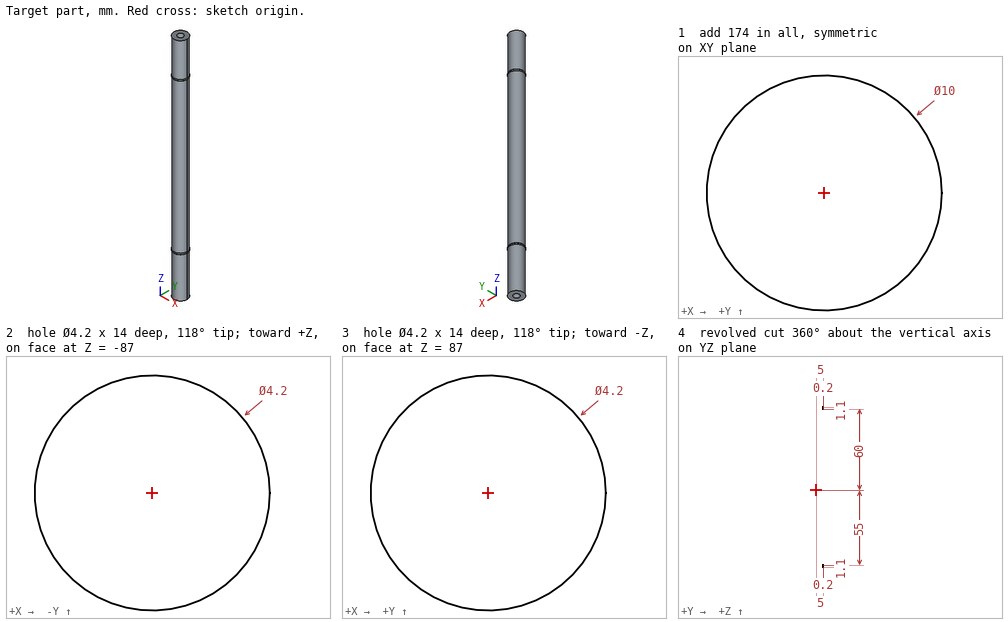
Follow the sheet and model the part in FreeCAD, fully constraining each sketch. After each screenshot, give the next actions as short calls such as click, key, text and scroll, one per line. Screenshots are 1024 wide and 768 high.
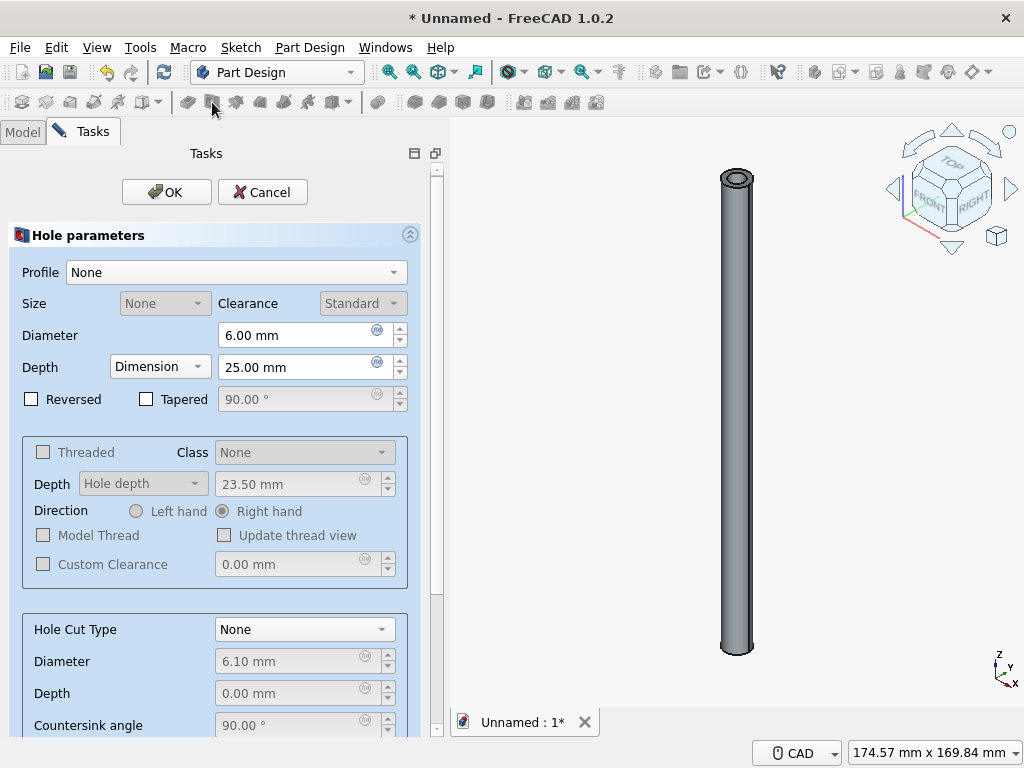
triple_click(305, 335)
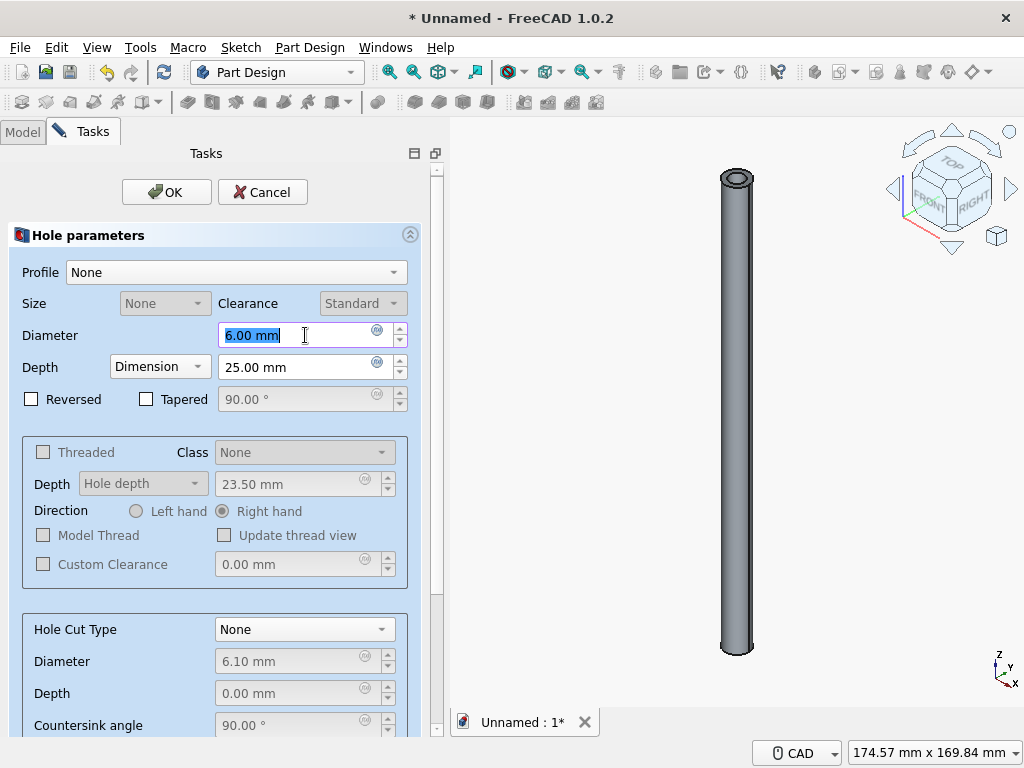
text(4.2)
key(Tab)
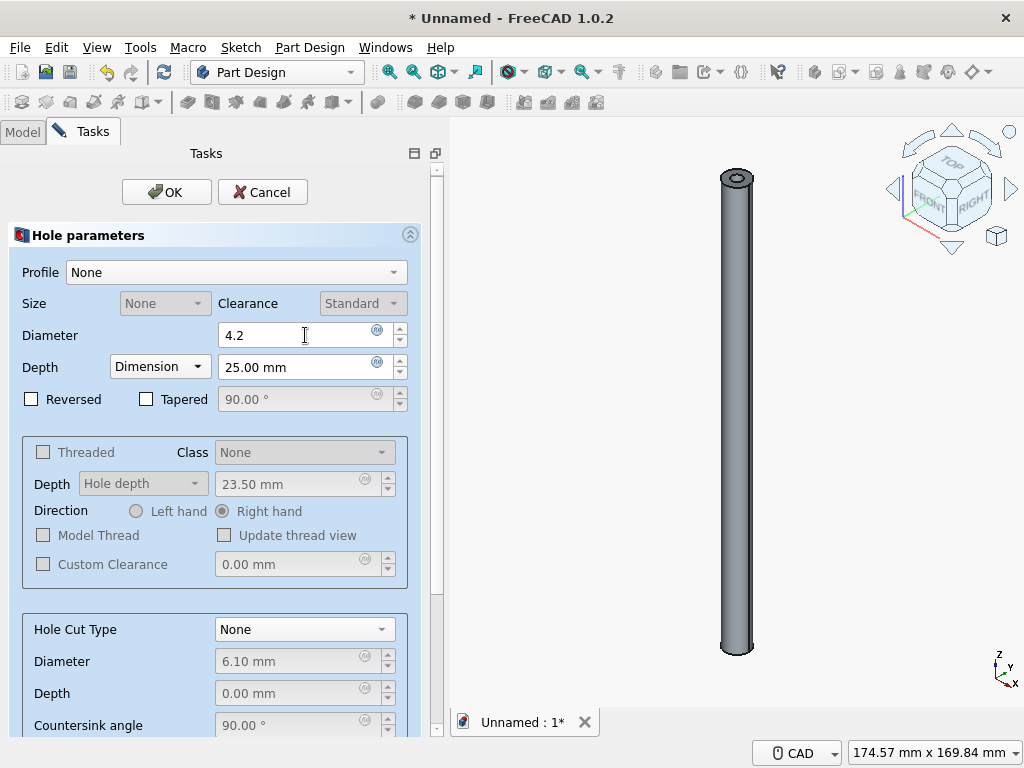
triple_click(305, 367)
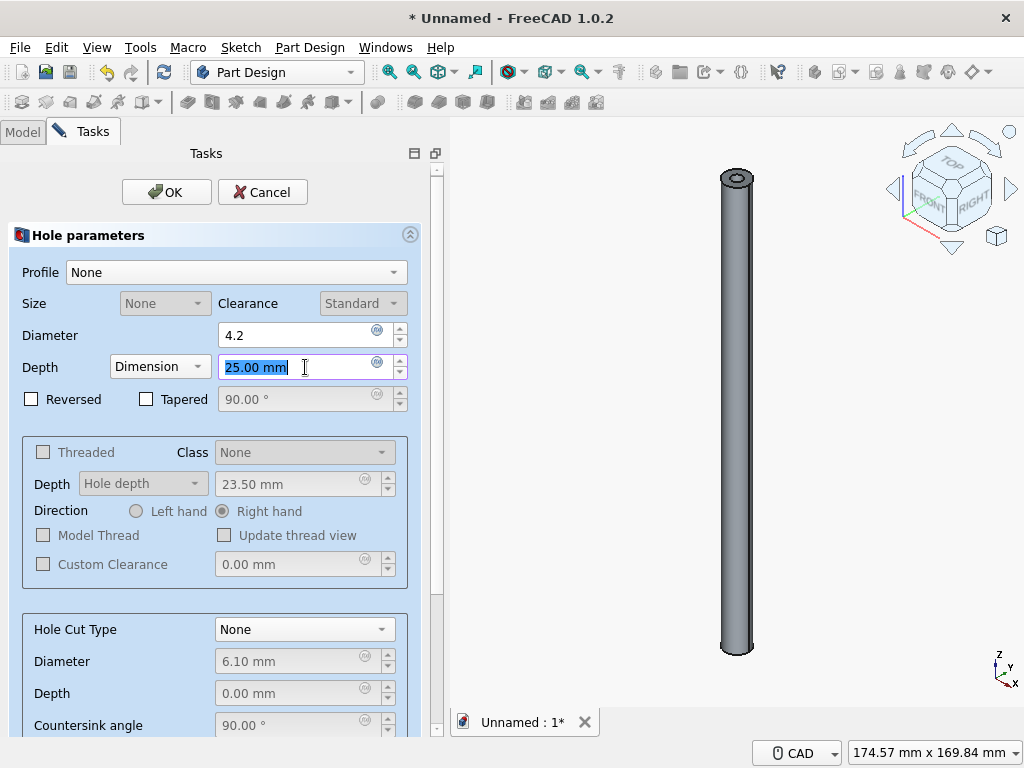
text(14)
key(Tab)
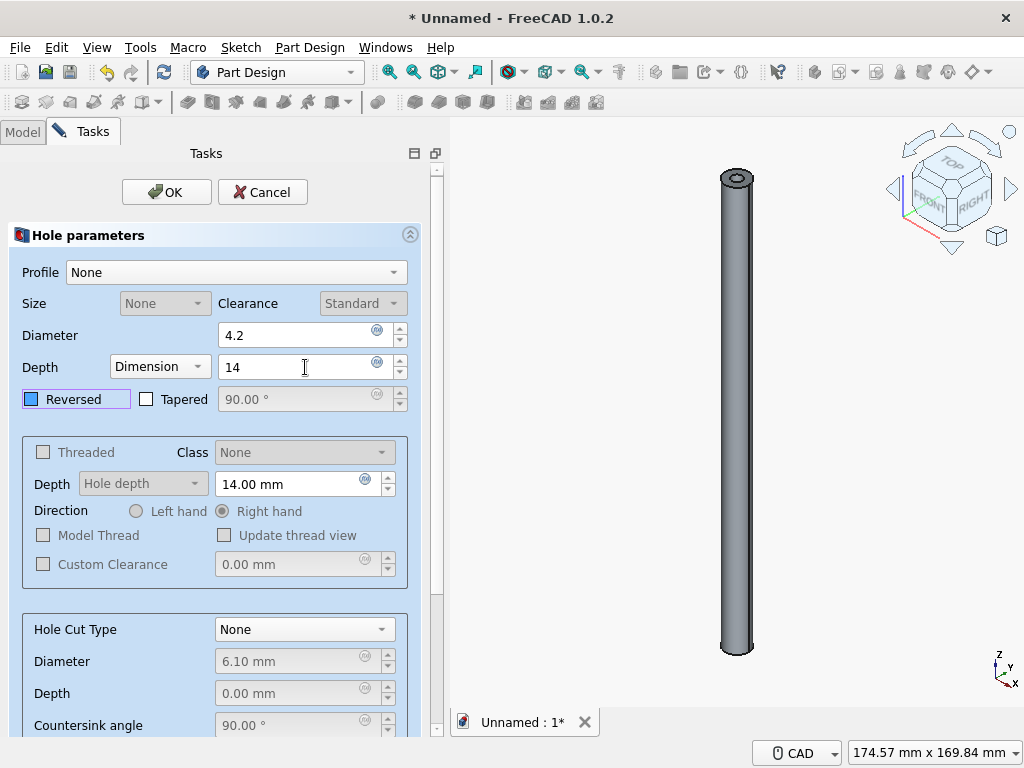
click(167, 192)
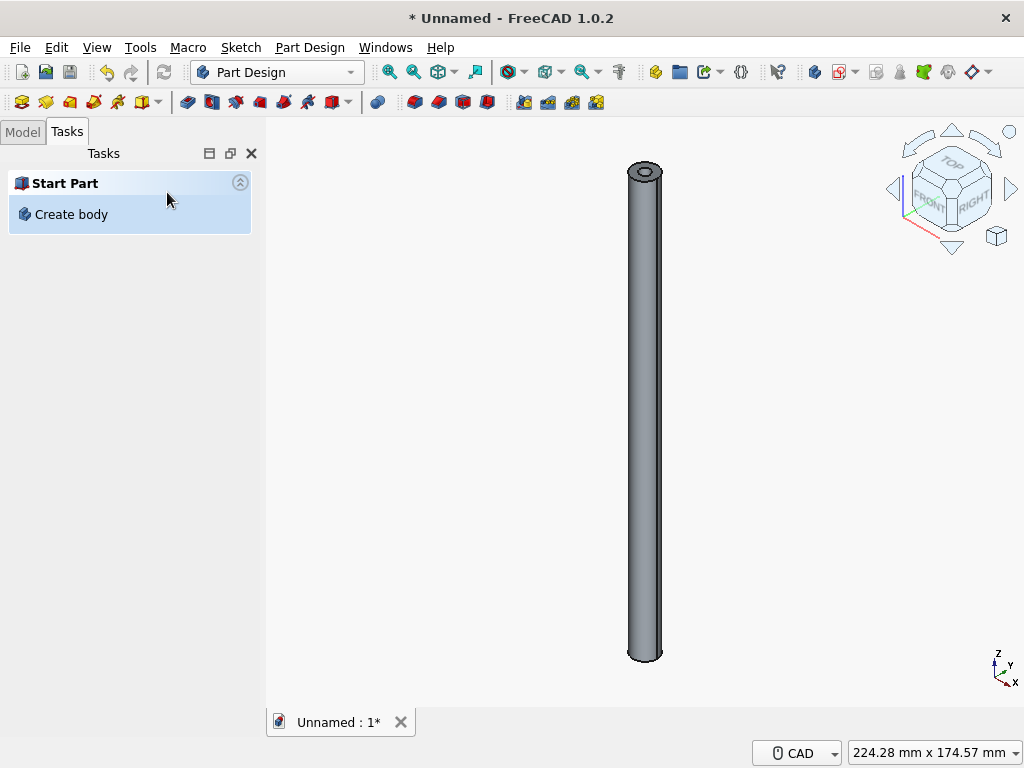
click(840, 72)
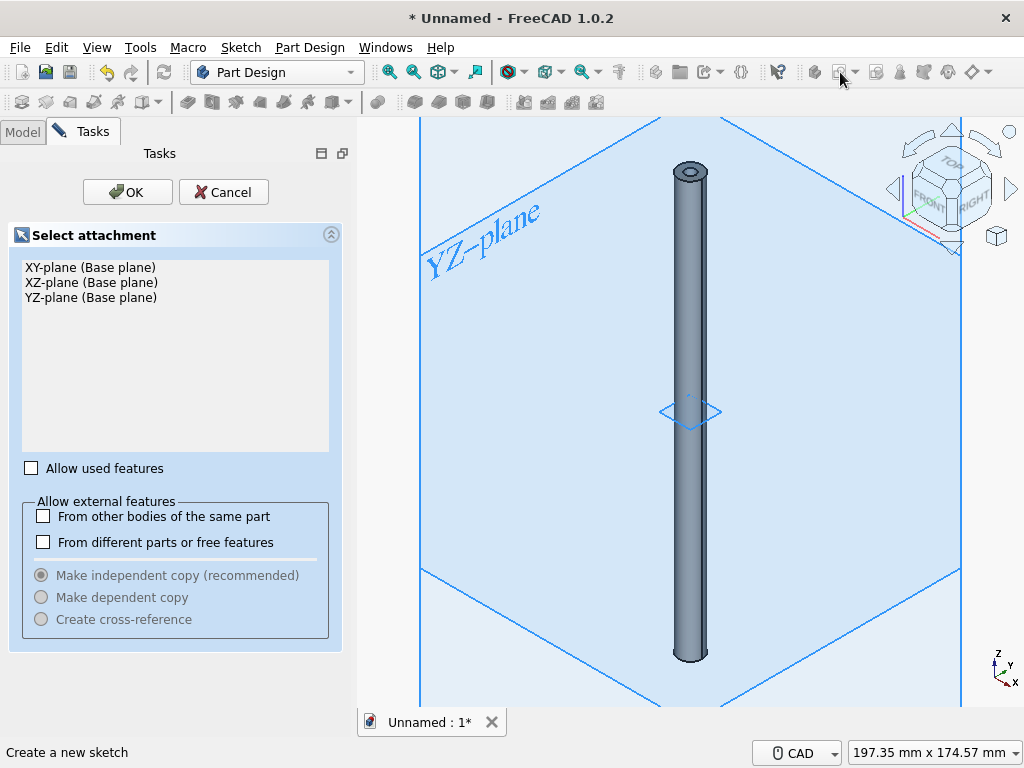
click(82, 298)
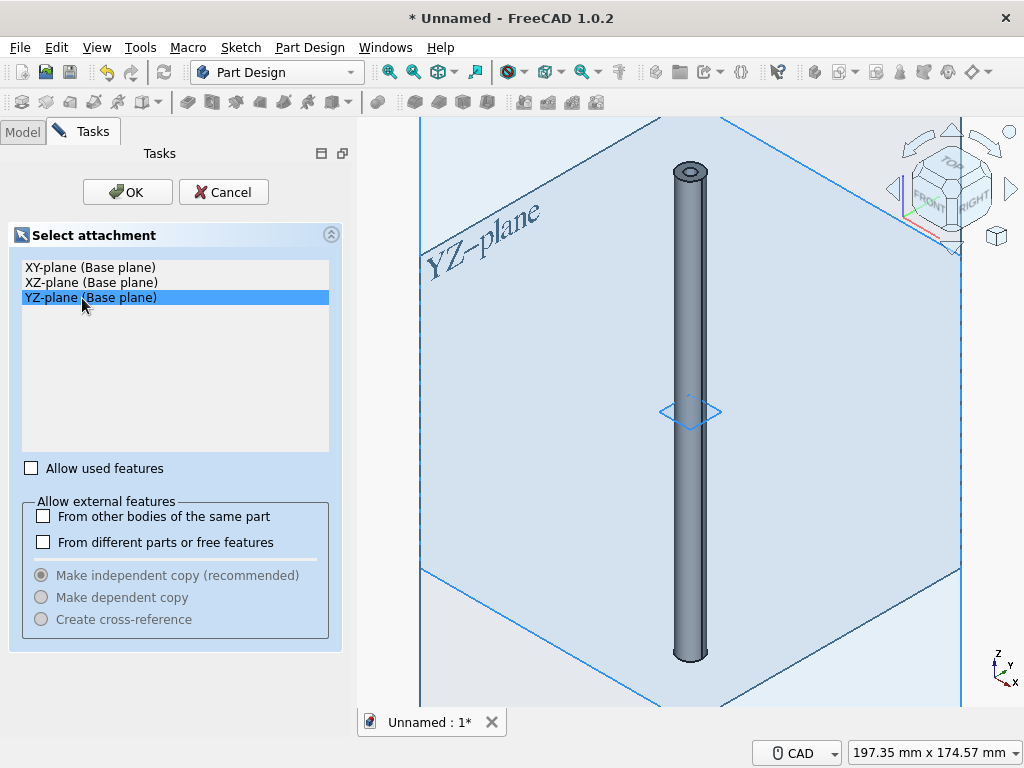
click(128, 192)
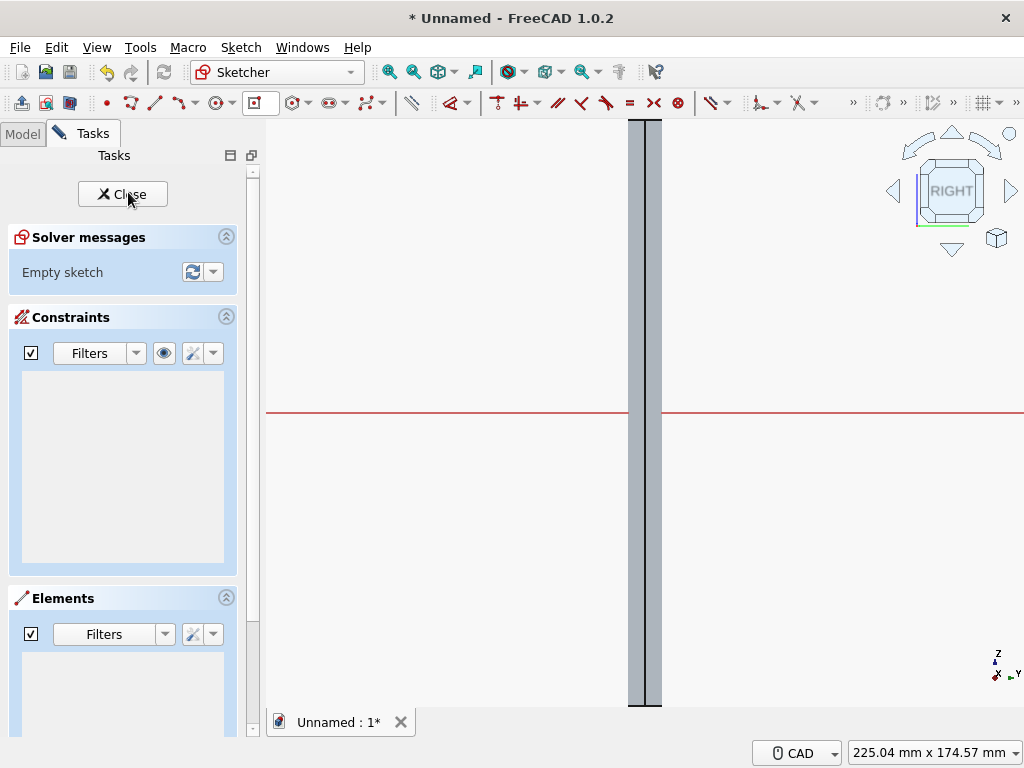
click(70, 104)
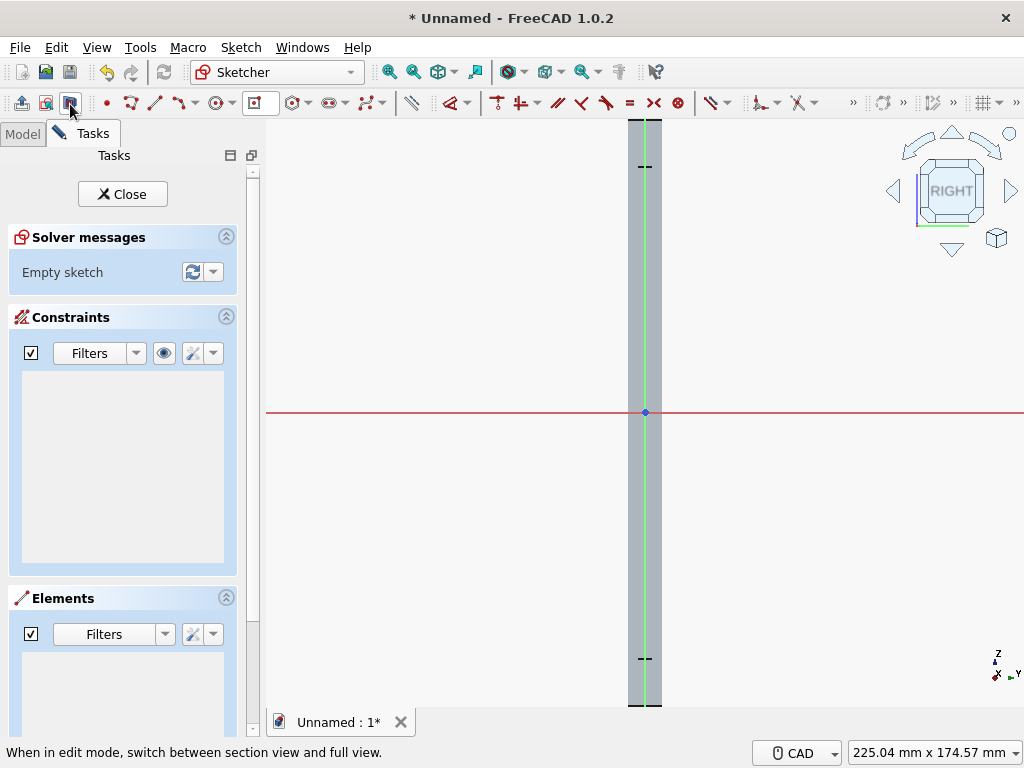
click(274, 104)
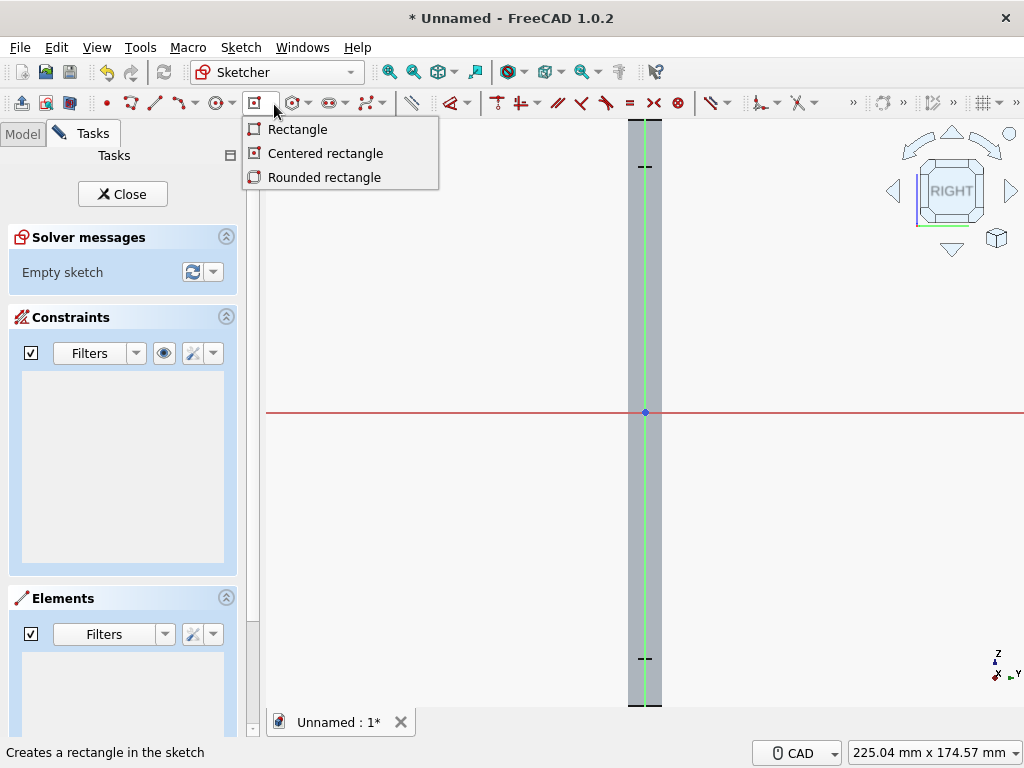
click(340, 129)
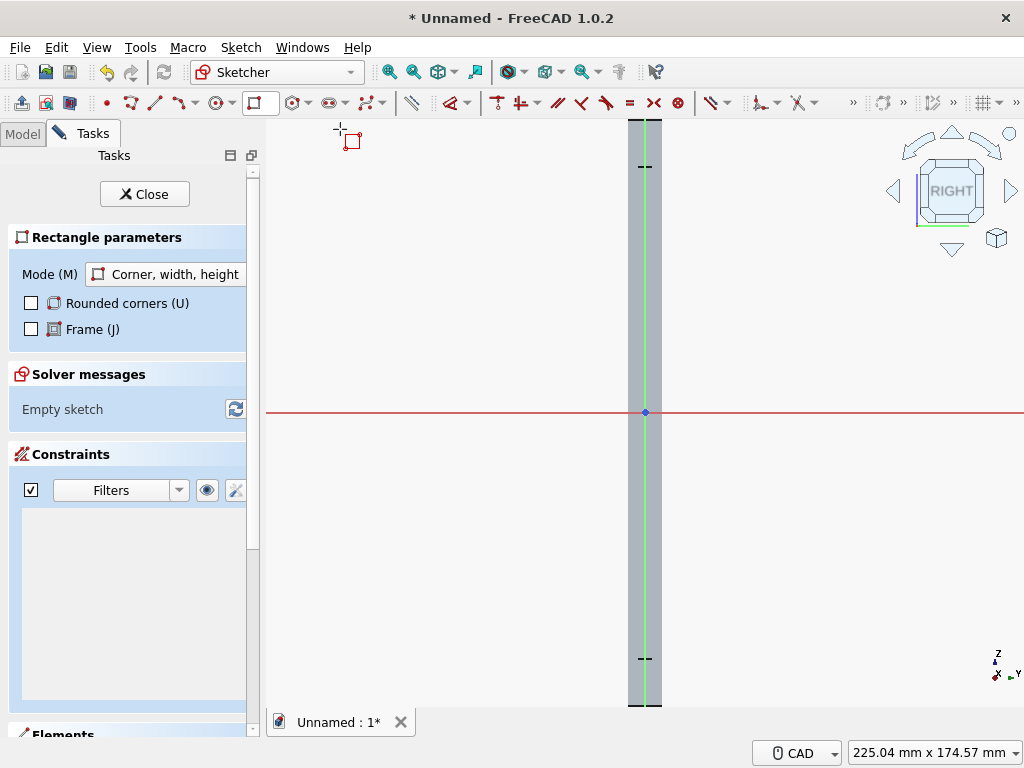
scroll(661, 207, up, 16)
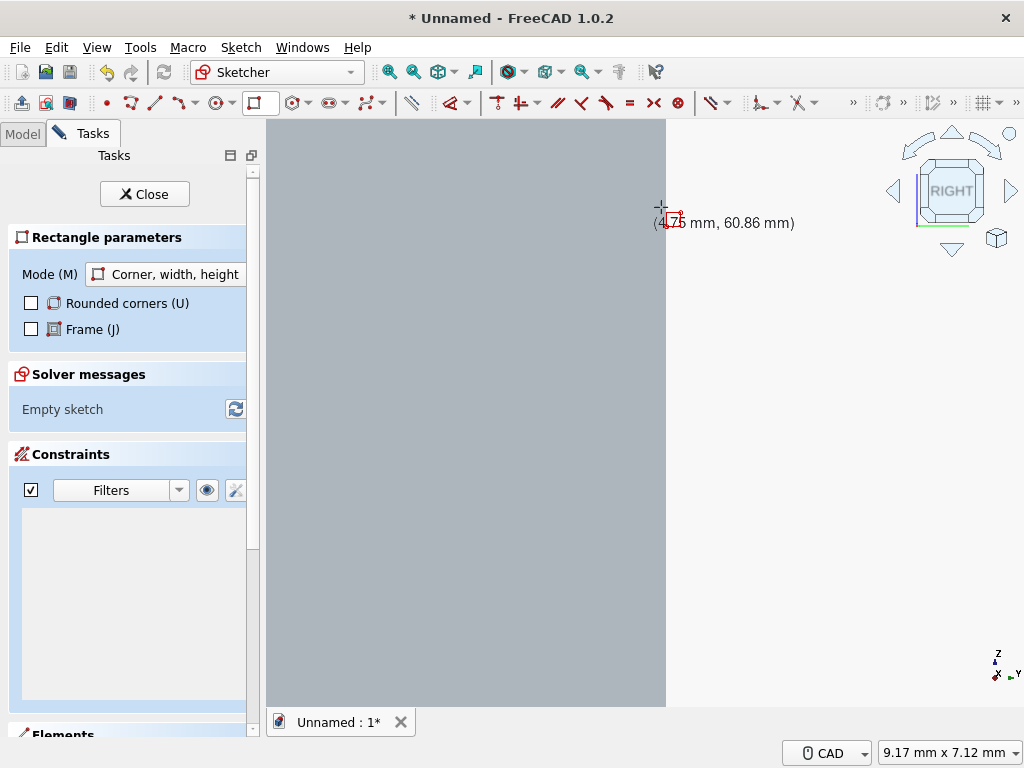
scroll(581, 216, down, 16)